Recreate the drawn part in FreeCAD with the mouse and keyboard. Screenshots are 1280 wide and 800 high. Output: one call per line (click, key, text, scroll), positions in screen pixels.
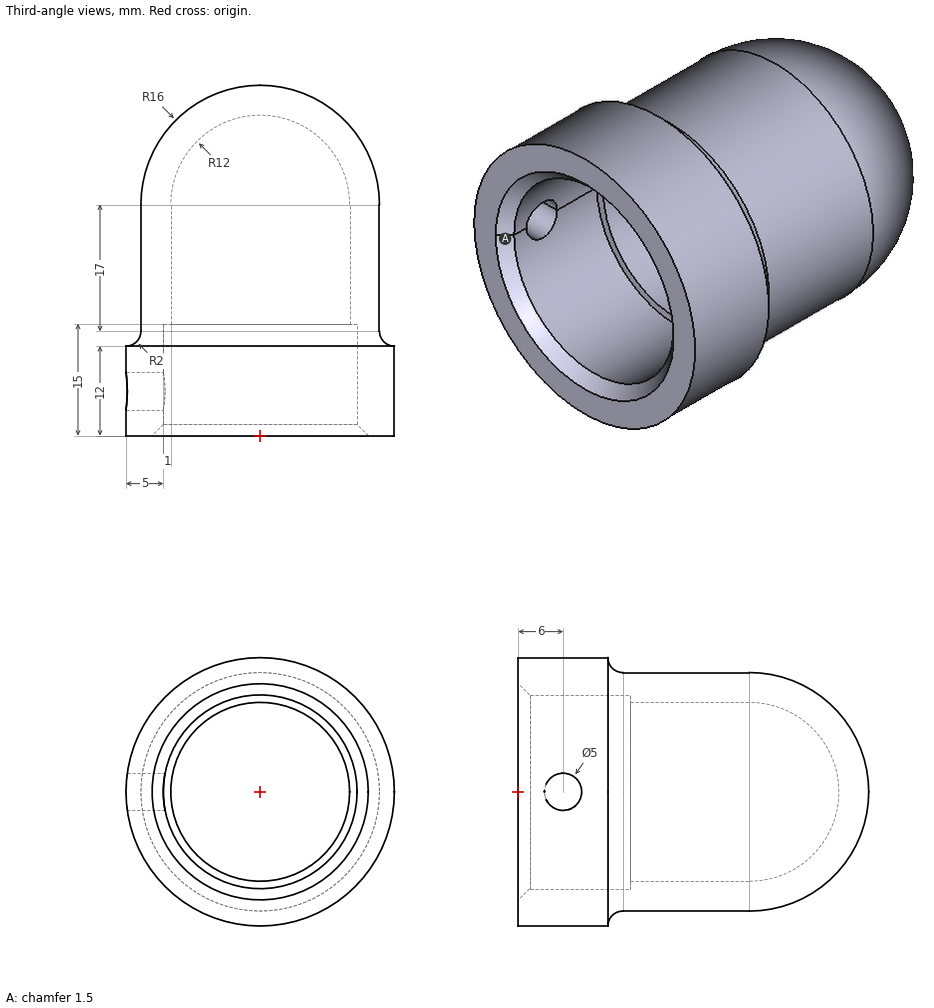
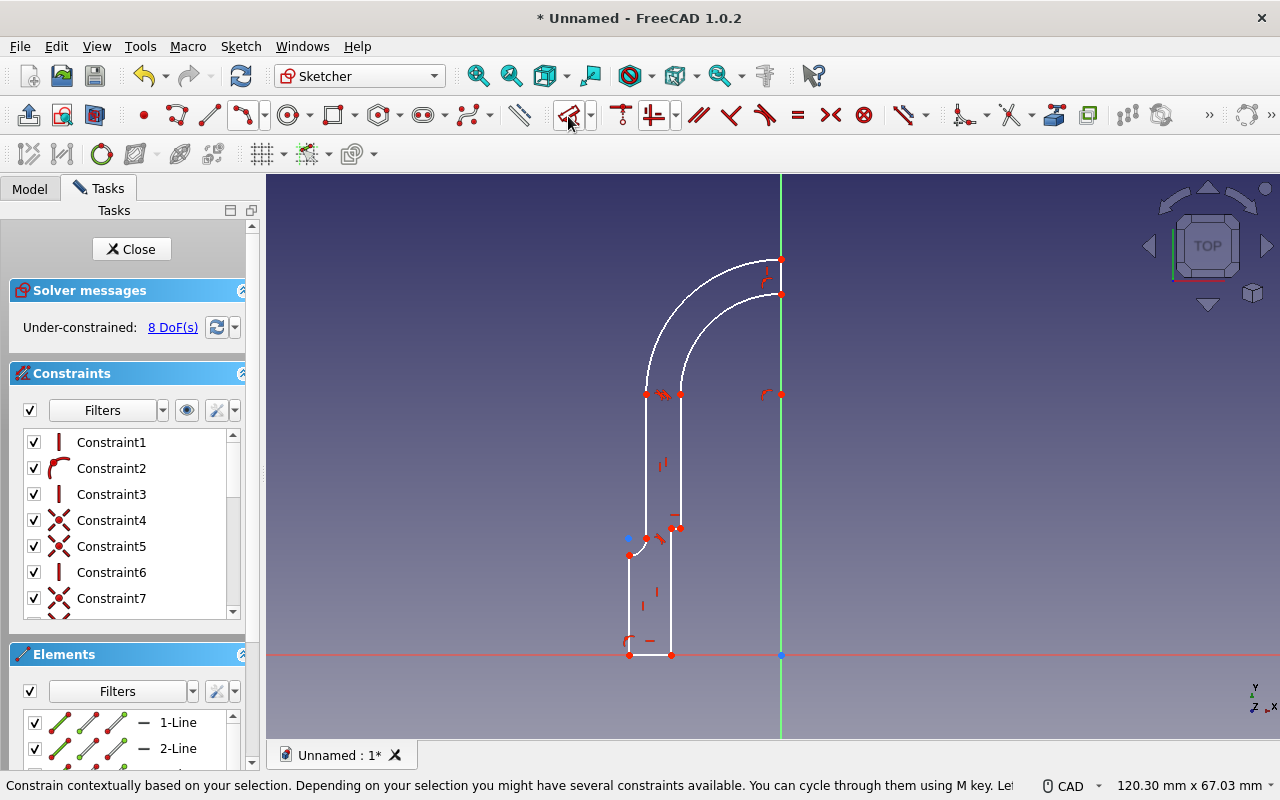
scroll(641, 551, up, 5)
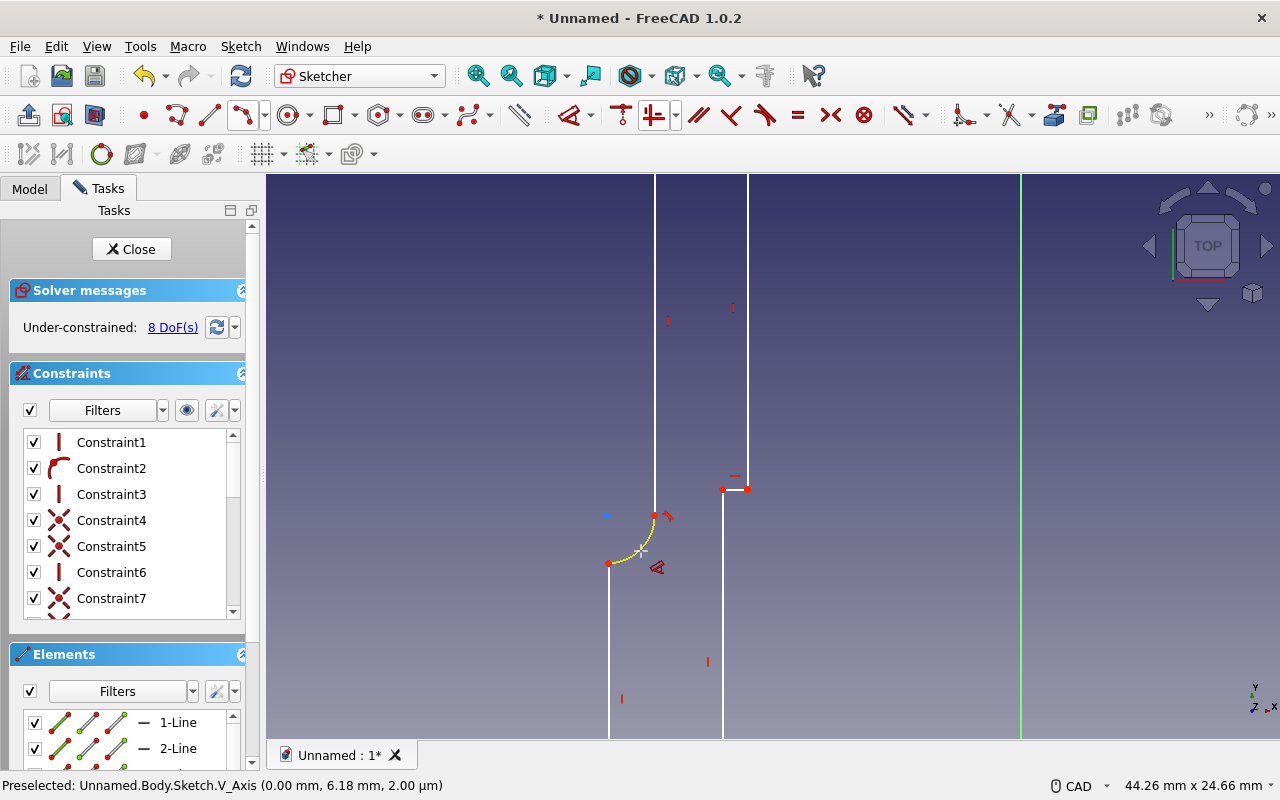
click(641, 549)
click(664, 571)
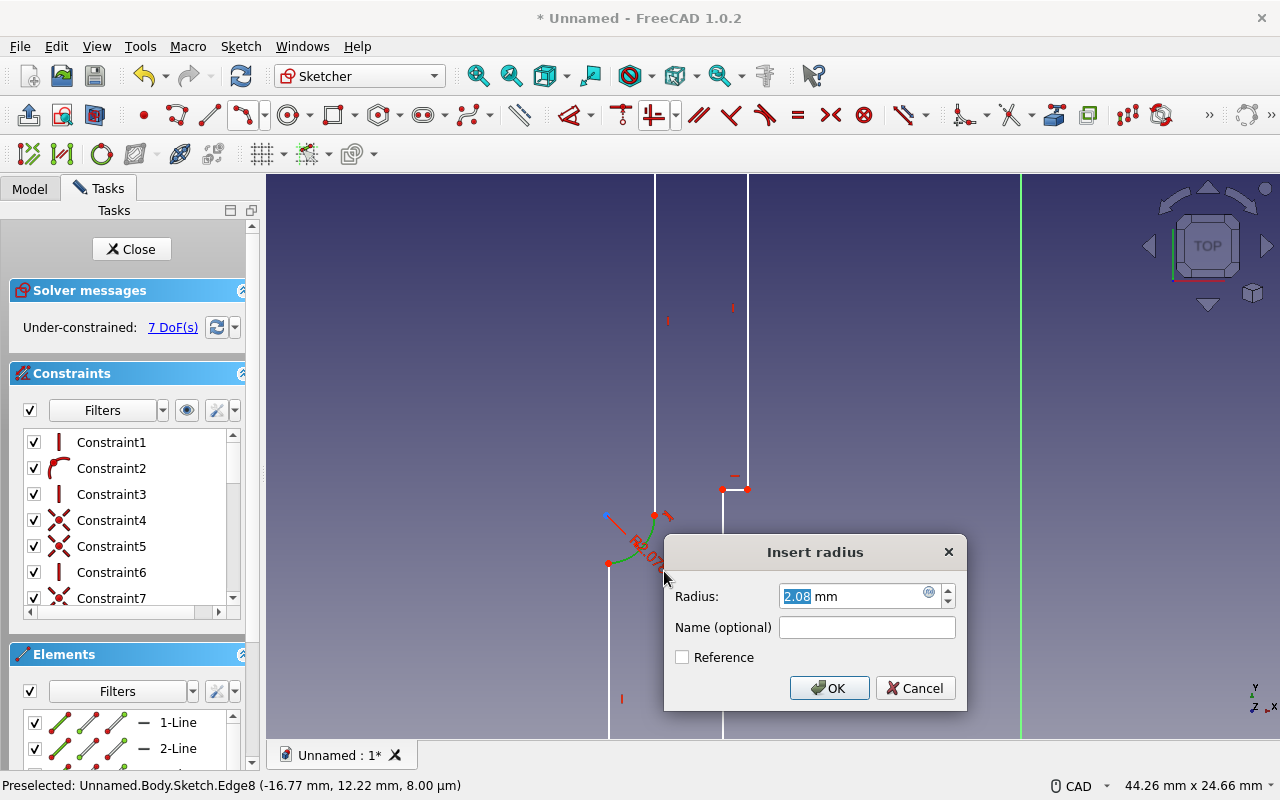
text(2)
key(Return)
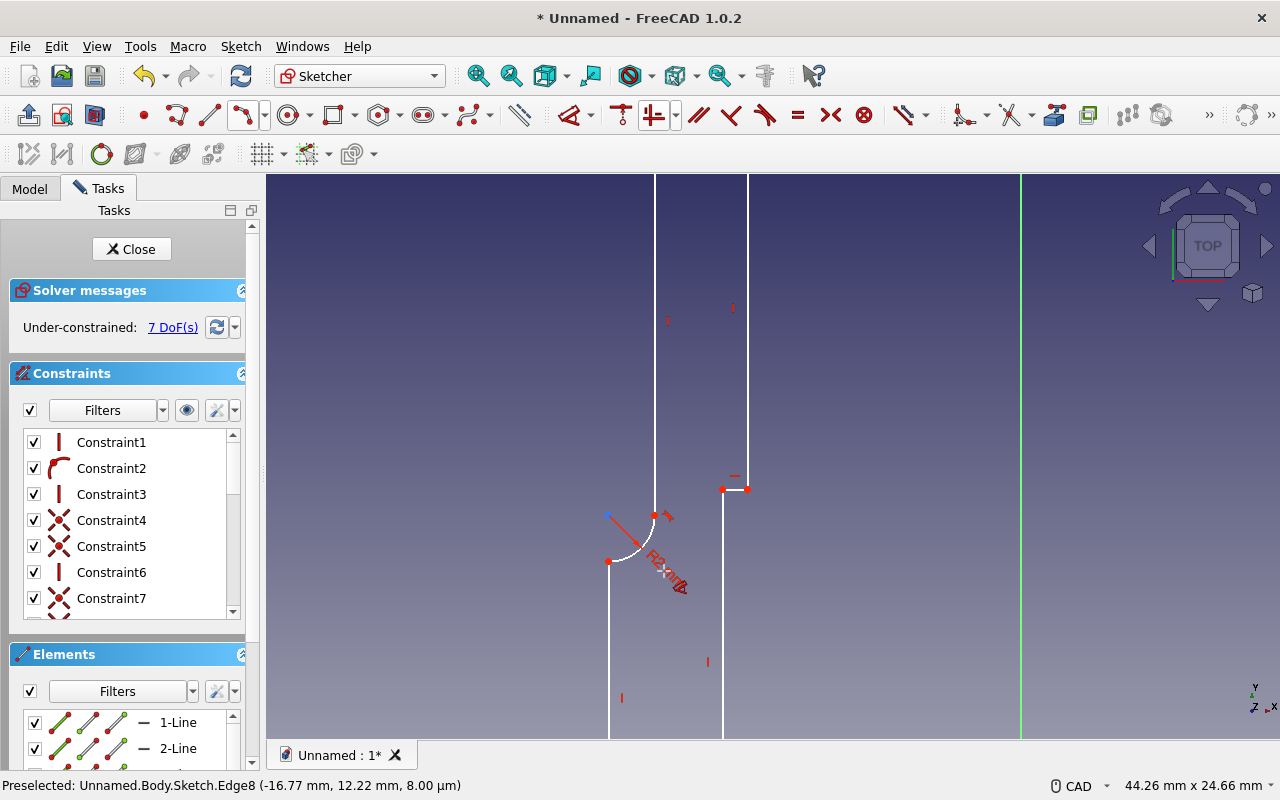
scroll(640, 551, down, 5)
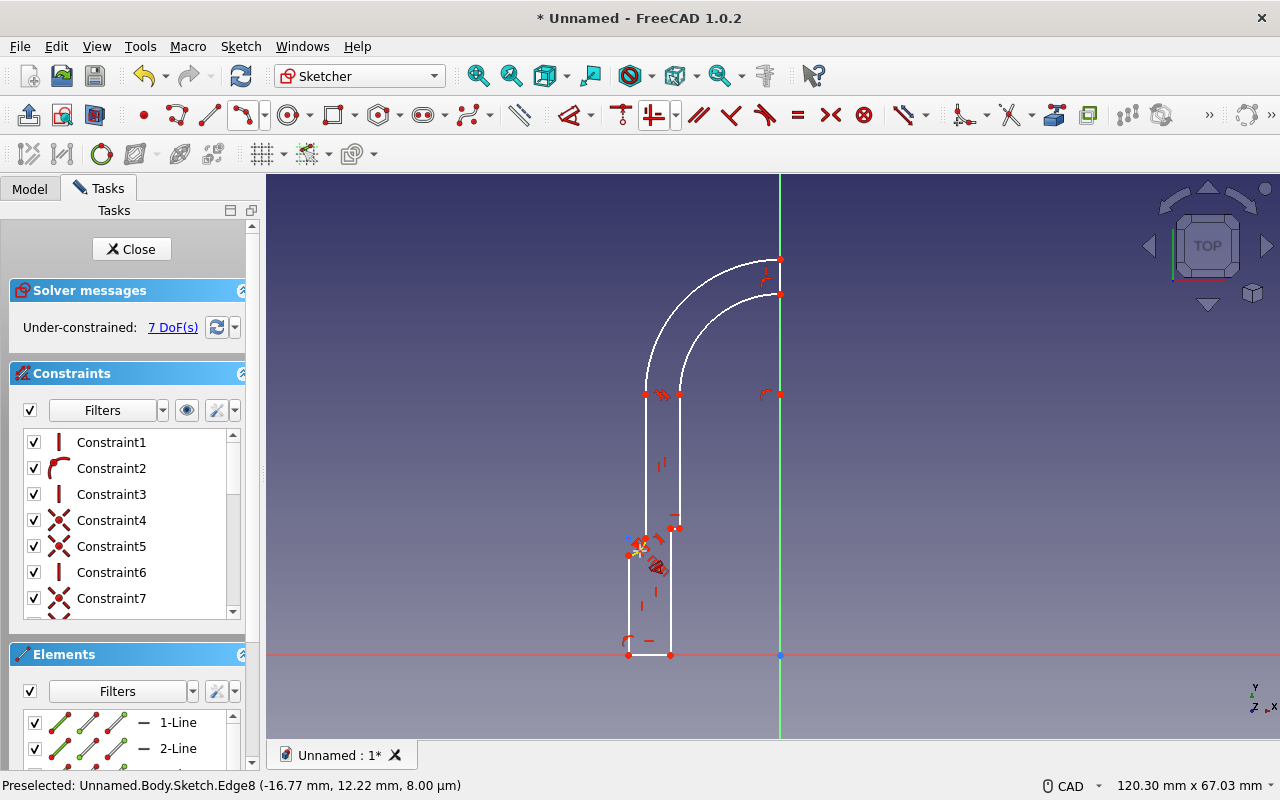
click(735, 305)
click(847, 280)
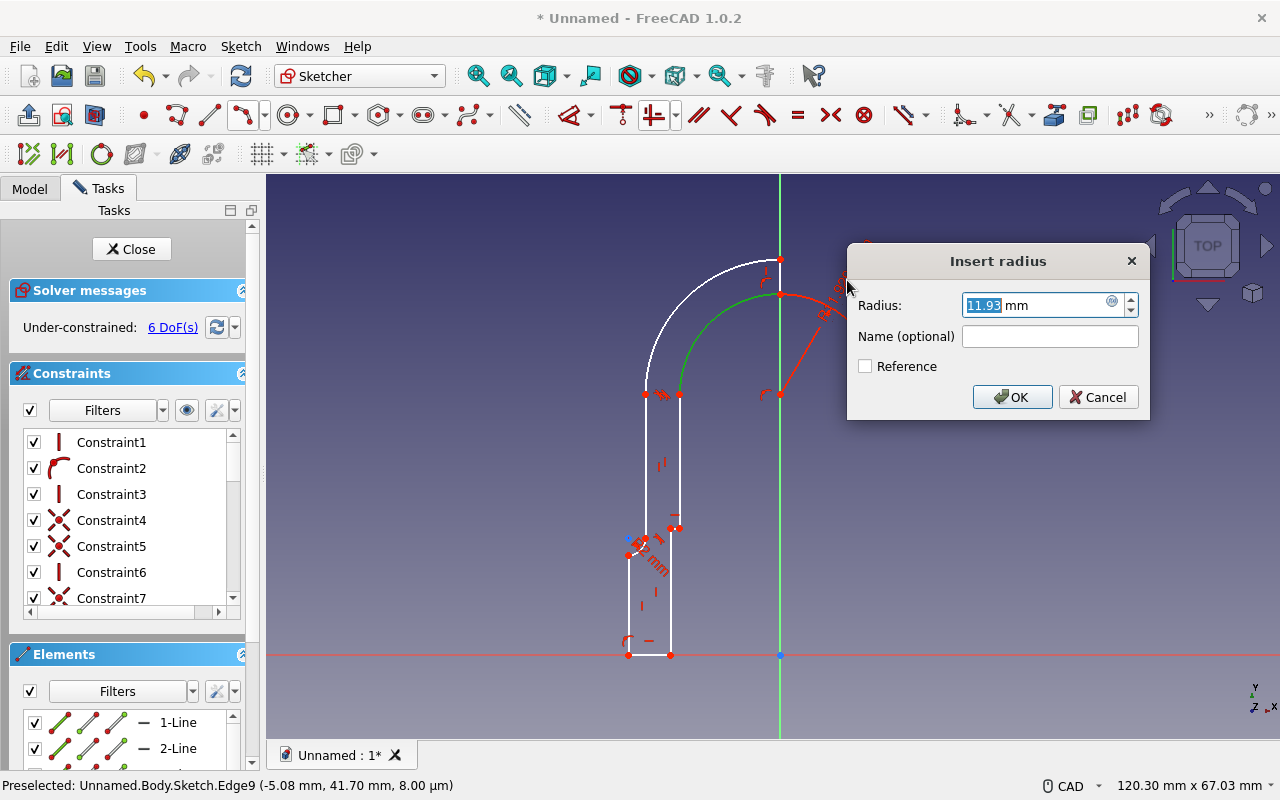
text(12)
key(Return)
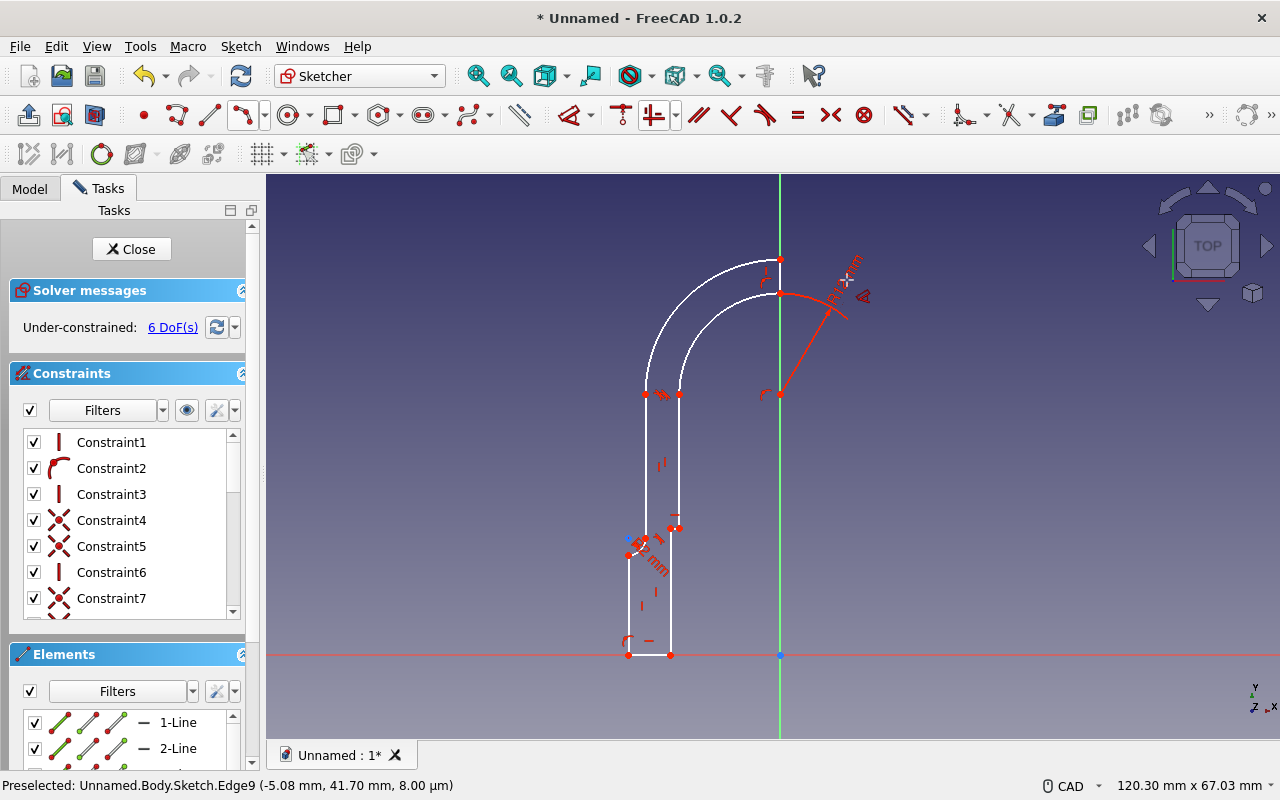
click(719, 274)
click(704, 245)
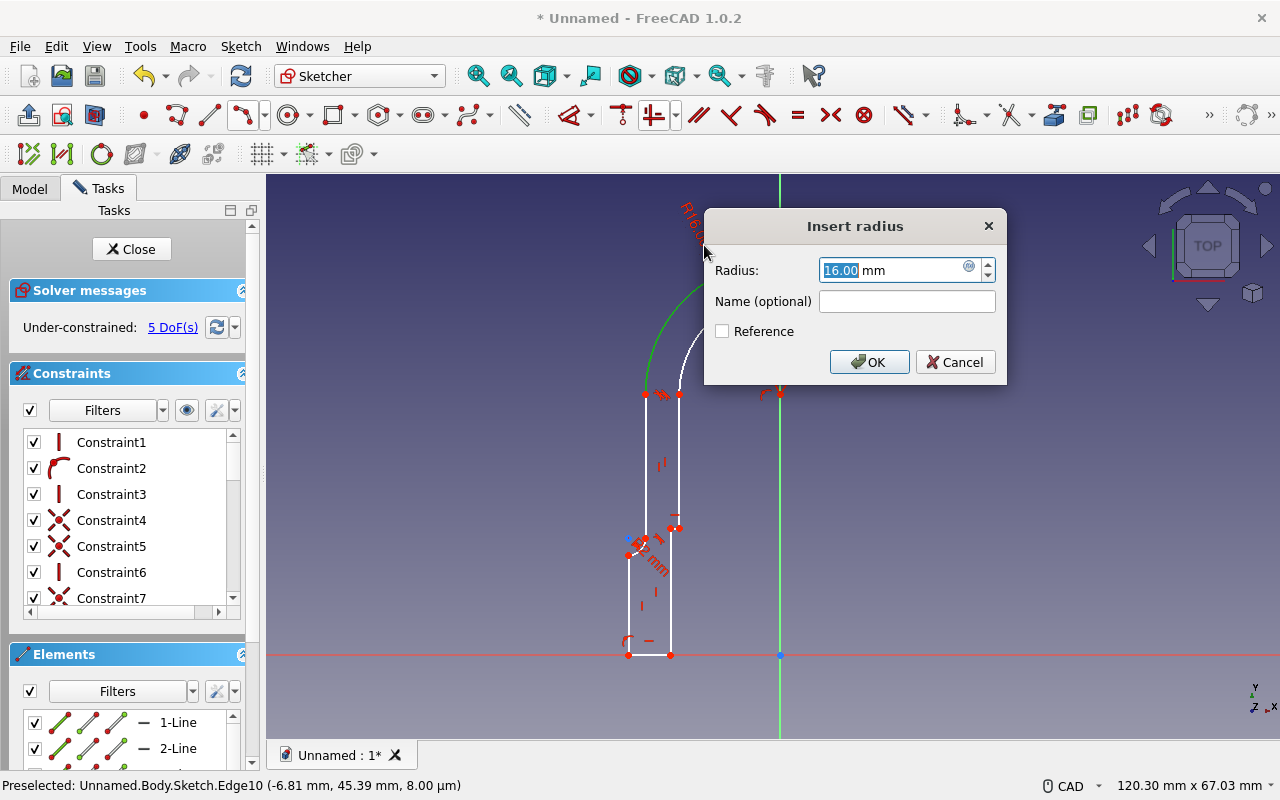
text(16)
key(Return)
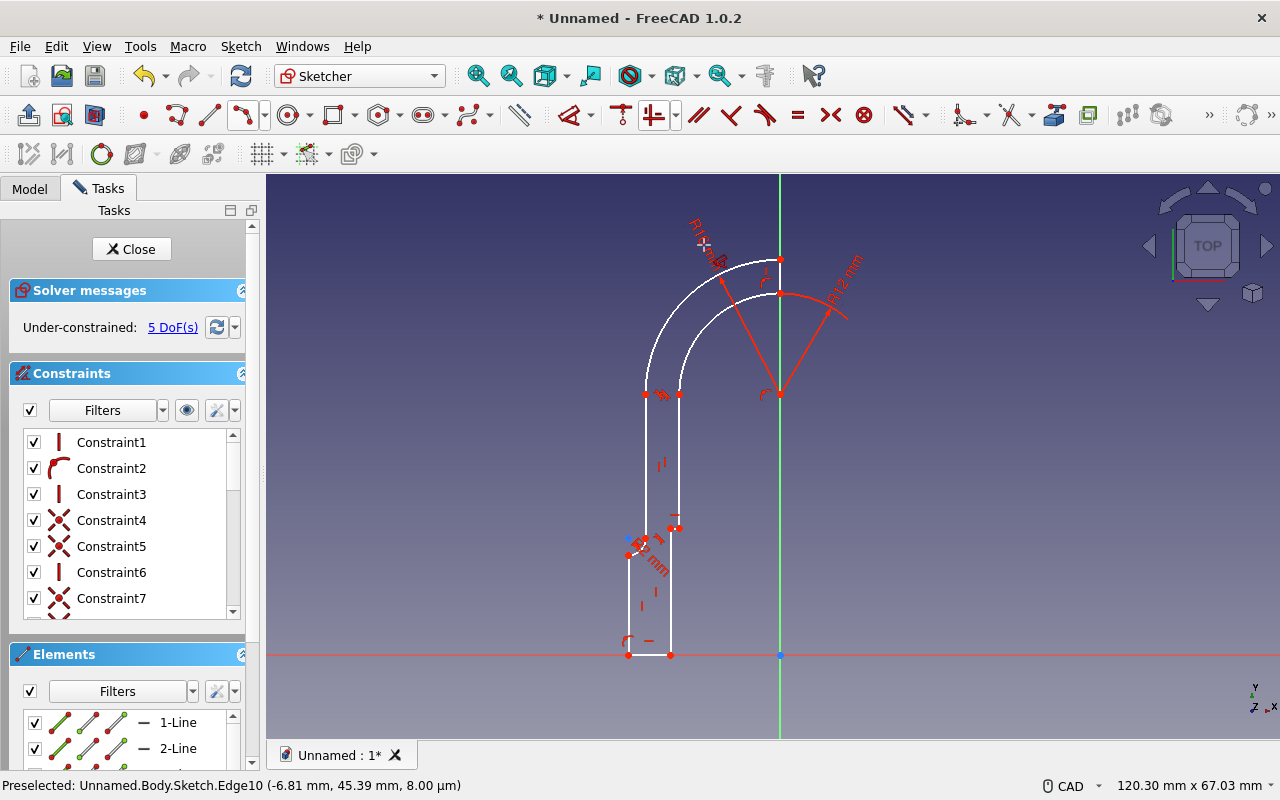
click(641, 655)
click(650, 689)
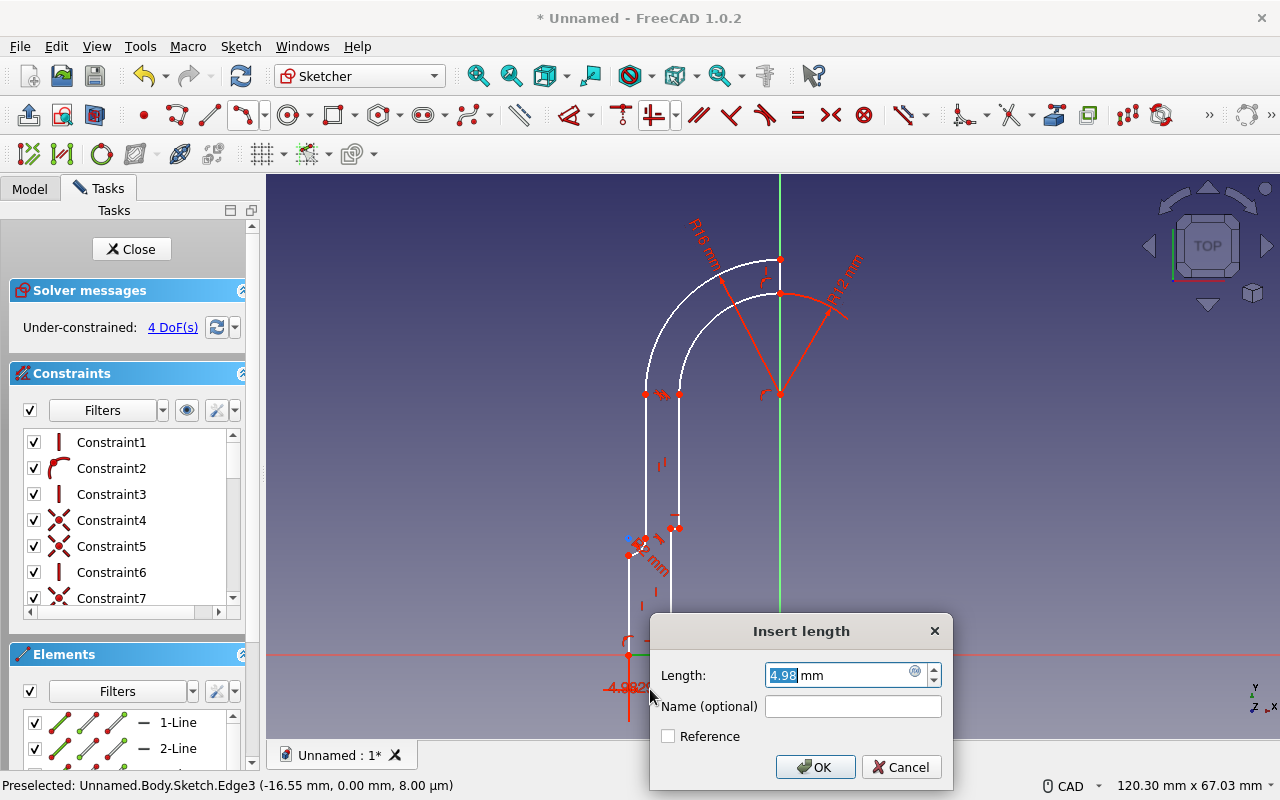
text(5)
key(Return)